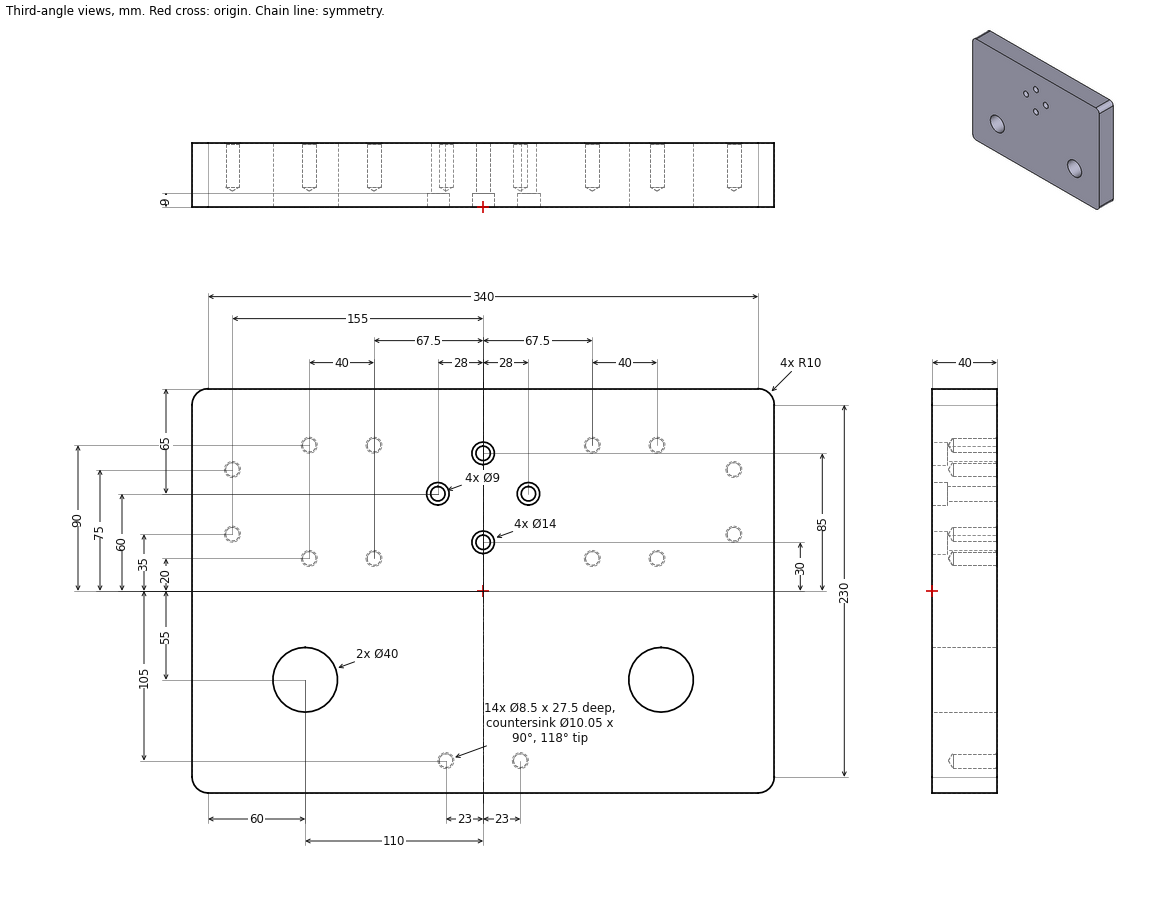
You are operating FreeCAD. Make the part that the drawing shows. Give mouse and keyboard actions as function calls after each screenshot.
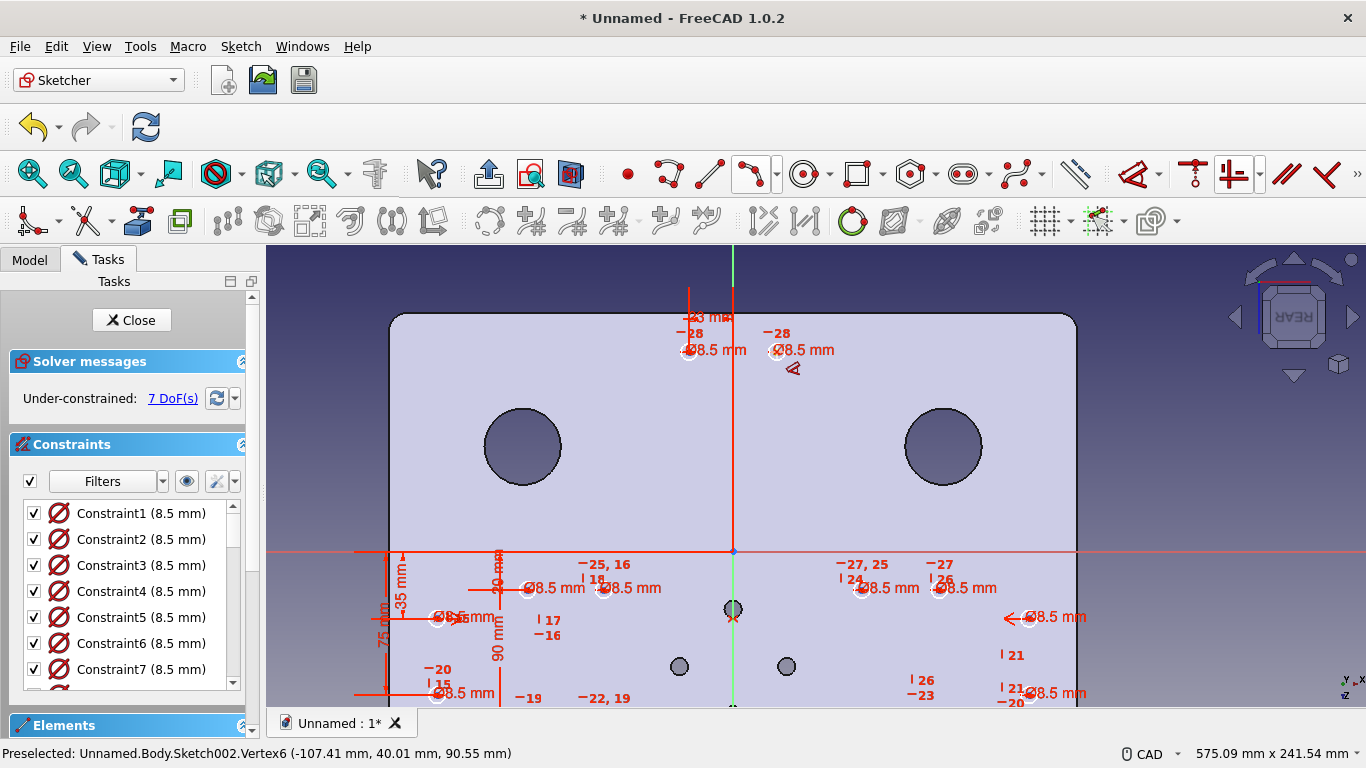
click(777, 352)
click(755, 586)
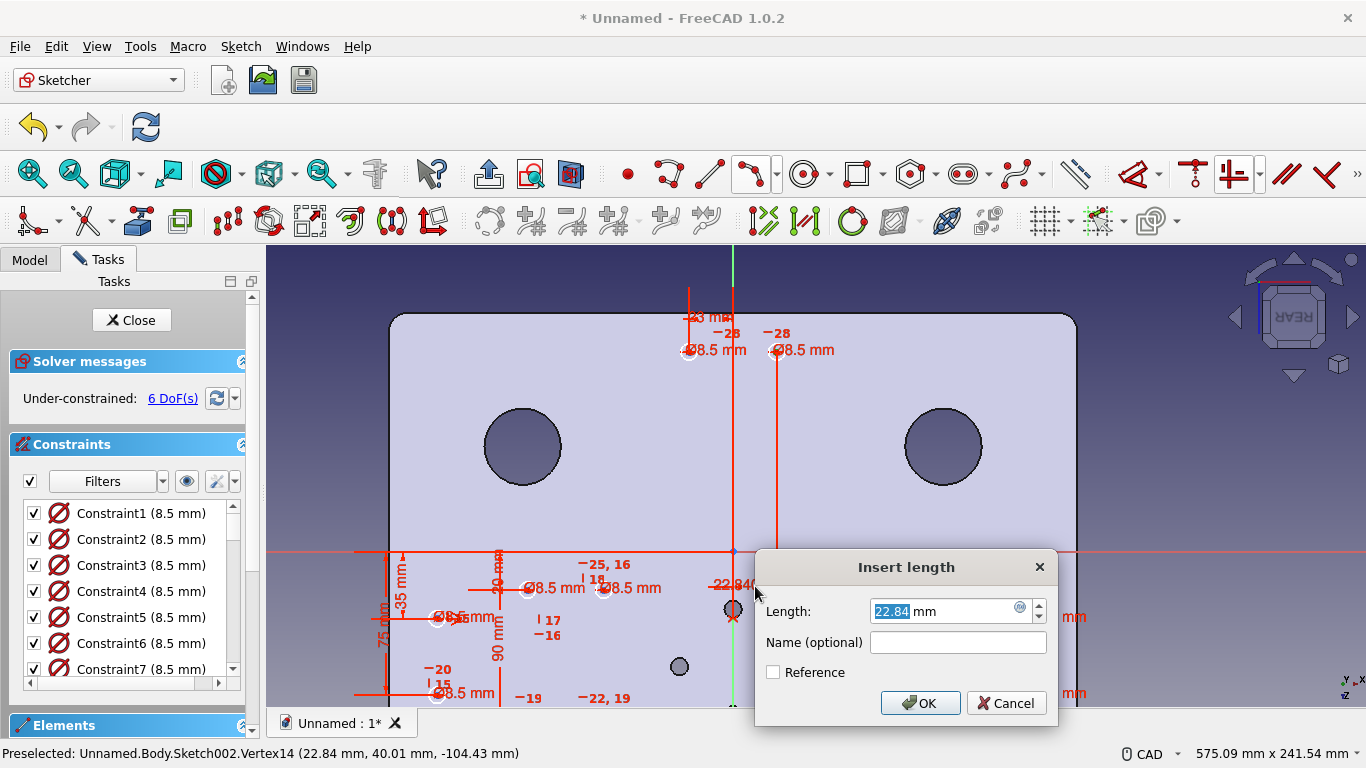
text(23)
key(Return)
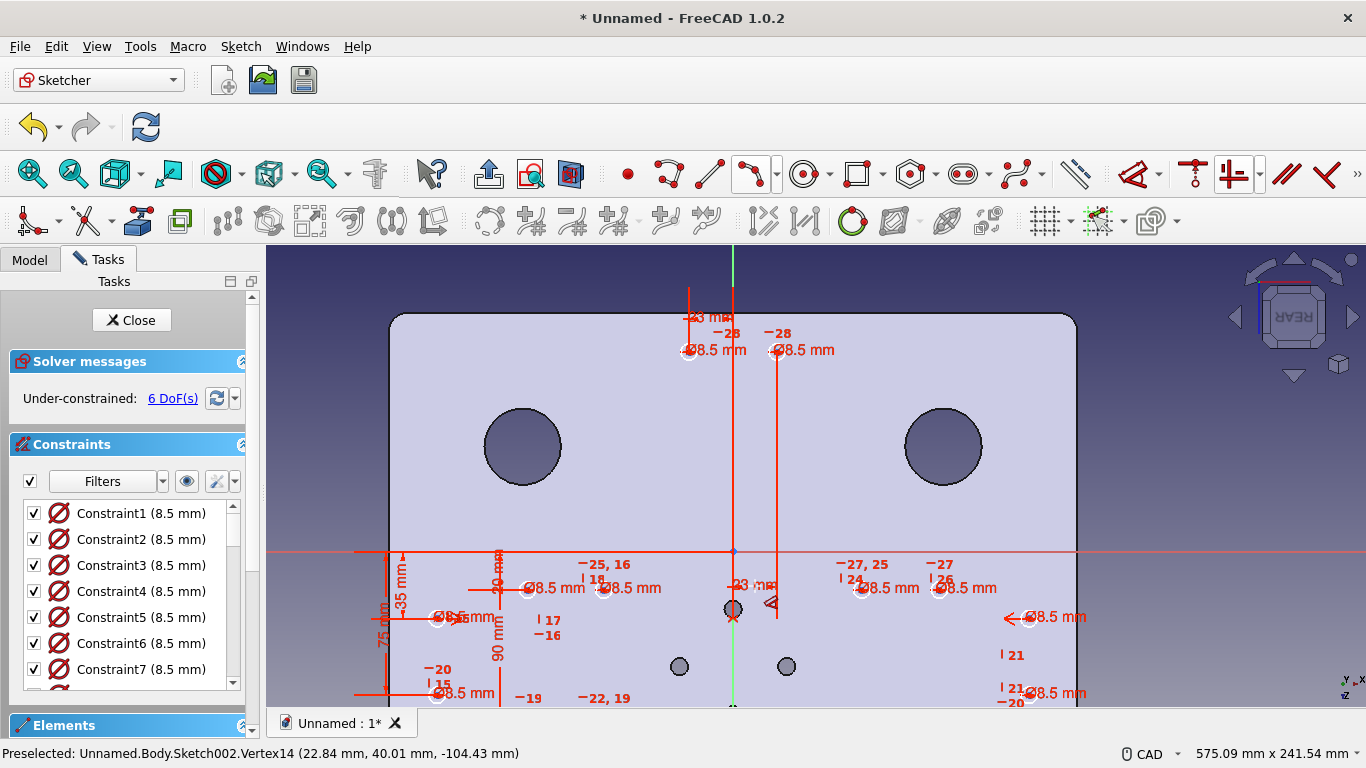
click(689, 352)
click(655, 452)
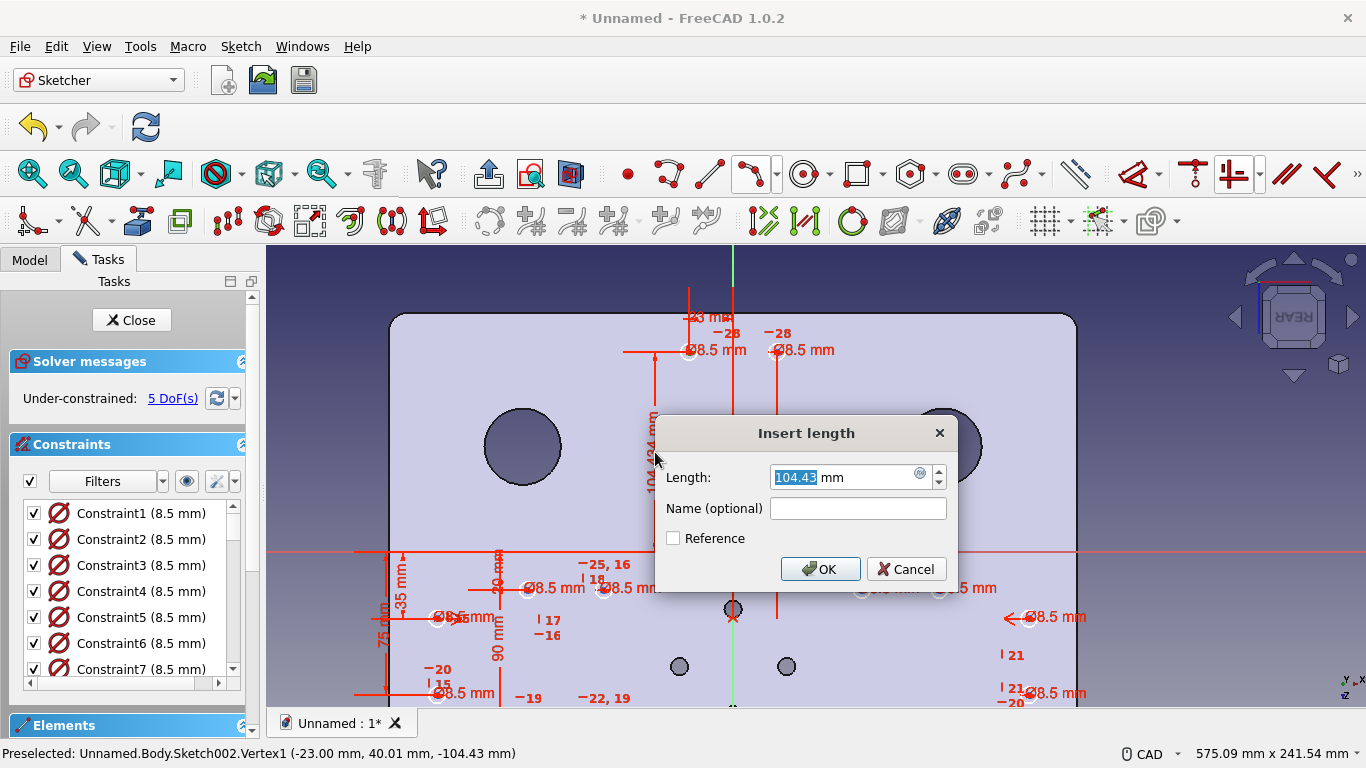
text(105)
key(Return)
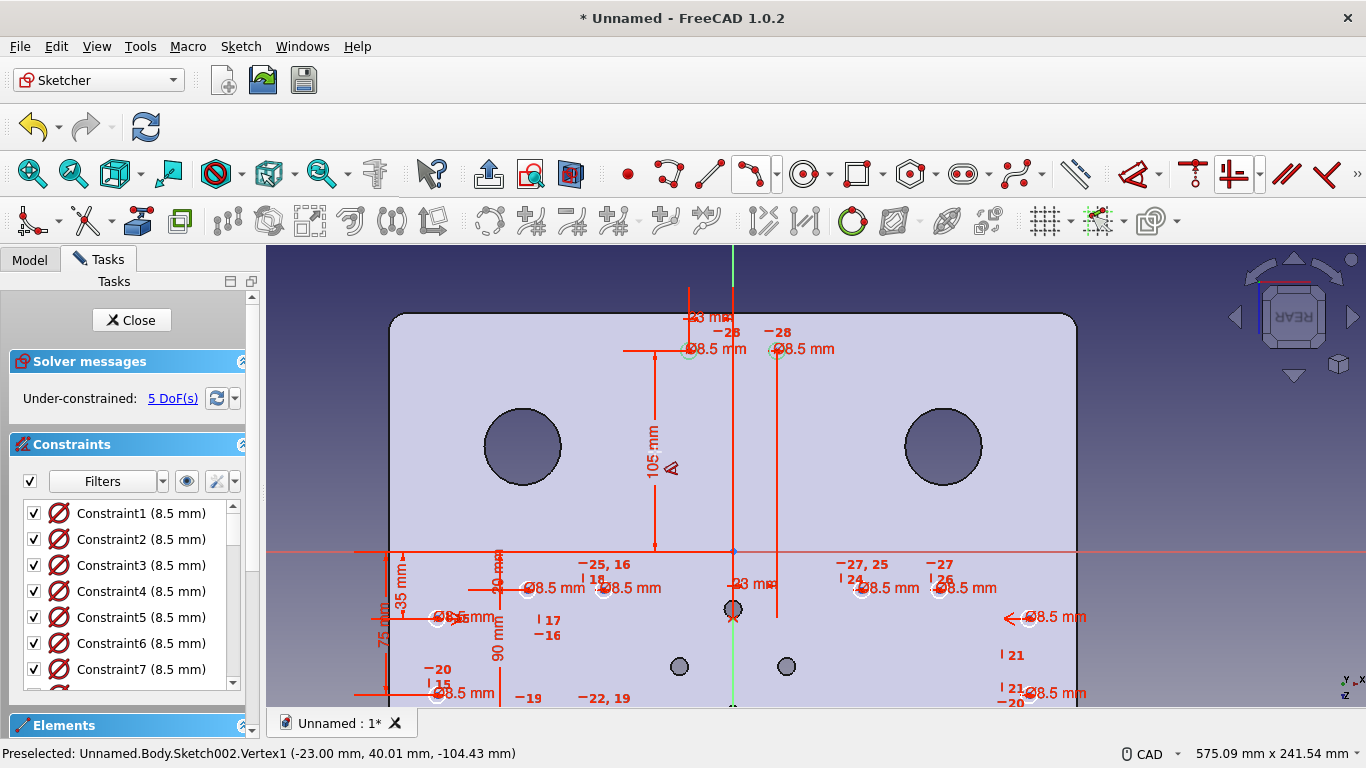
click(437, 619)
click(585, 653)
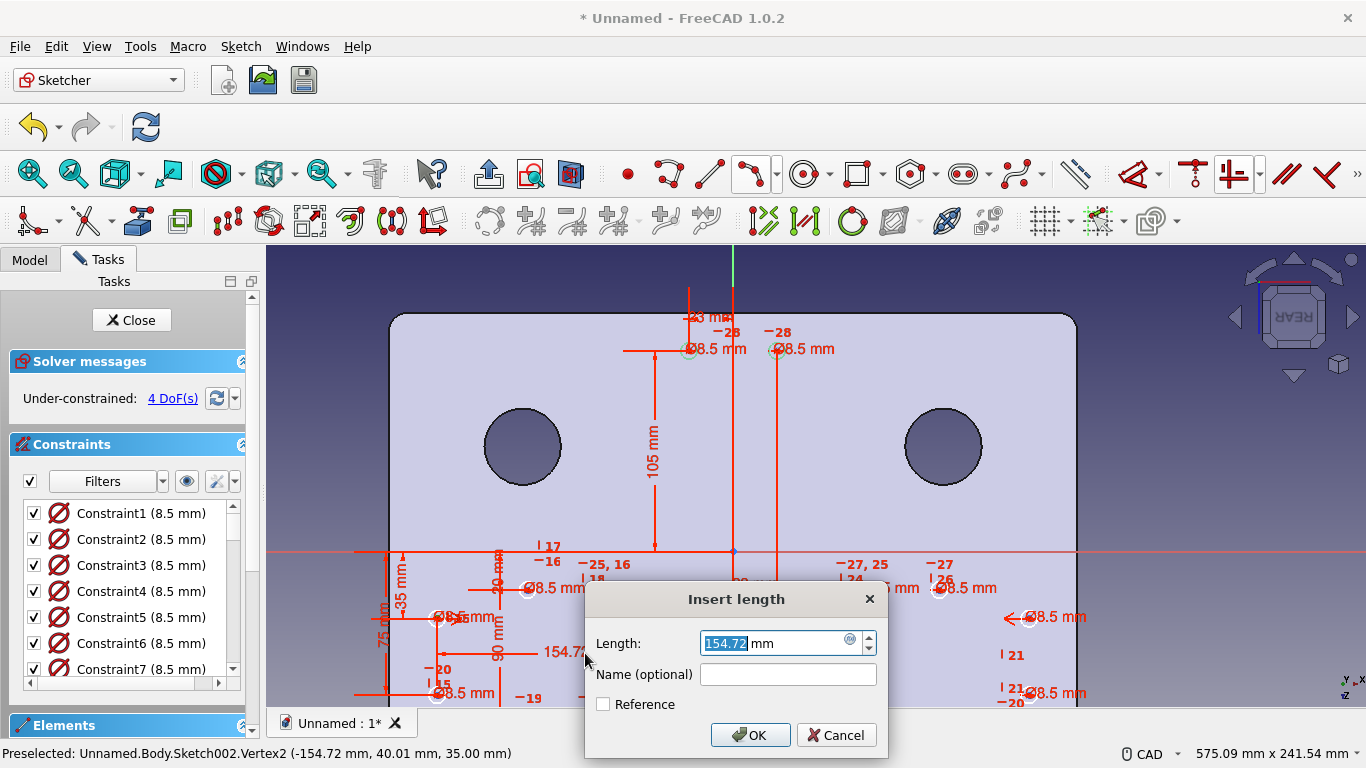
text(155)
key(Return)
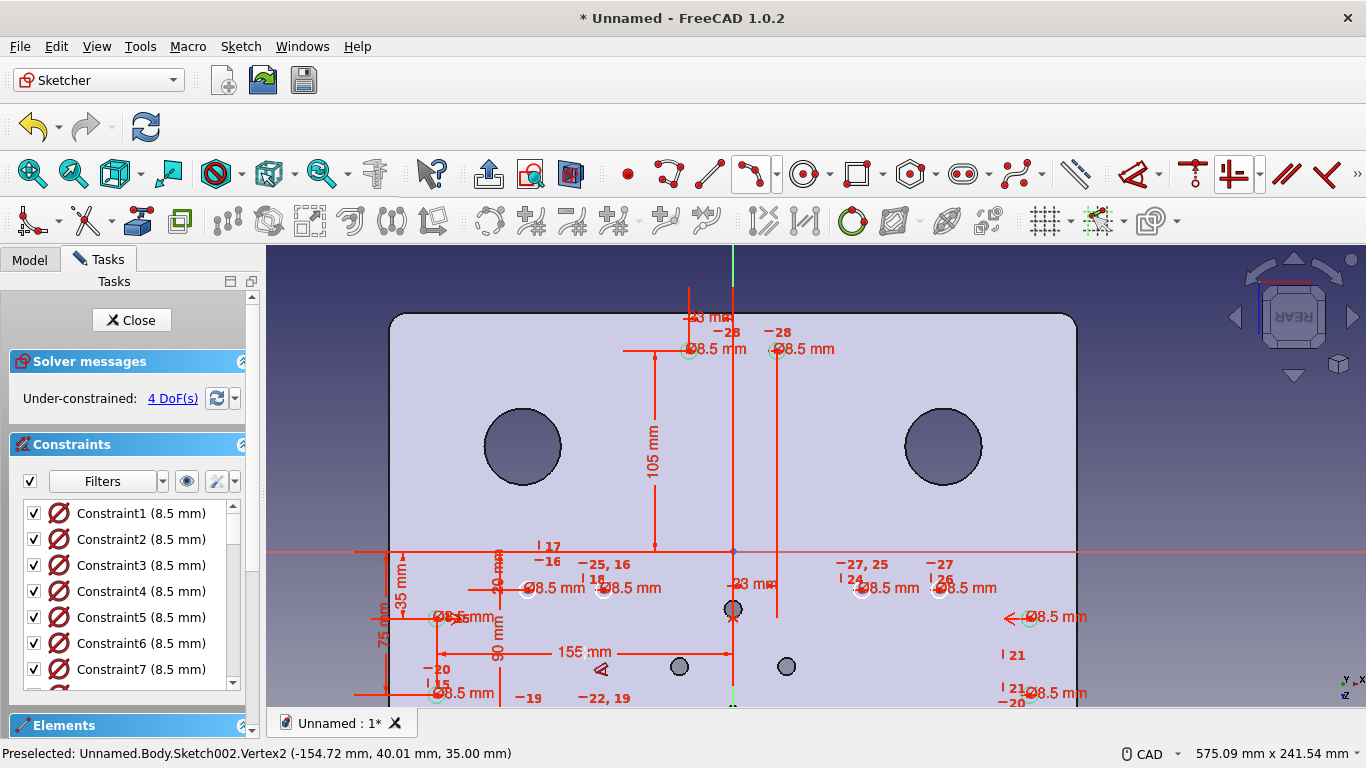
click(528, 590)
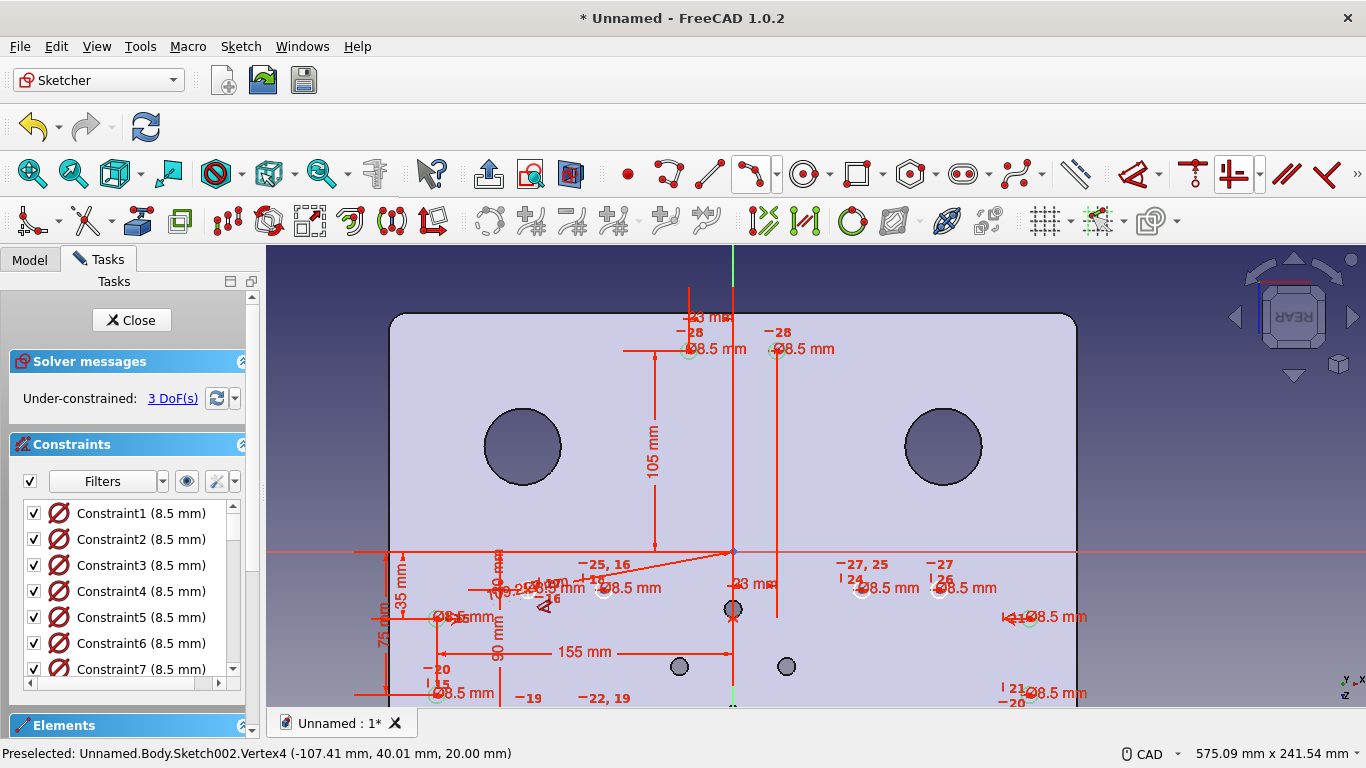
click(604, 590)
click(583, 624)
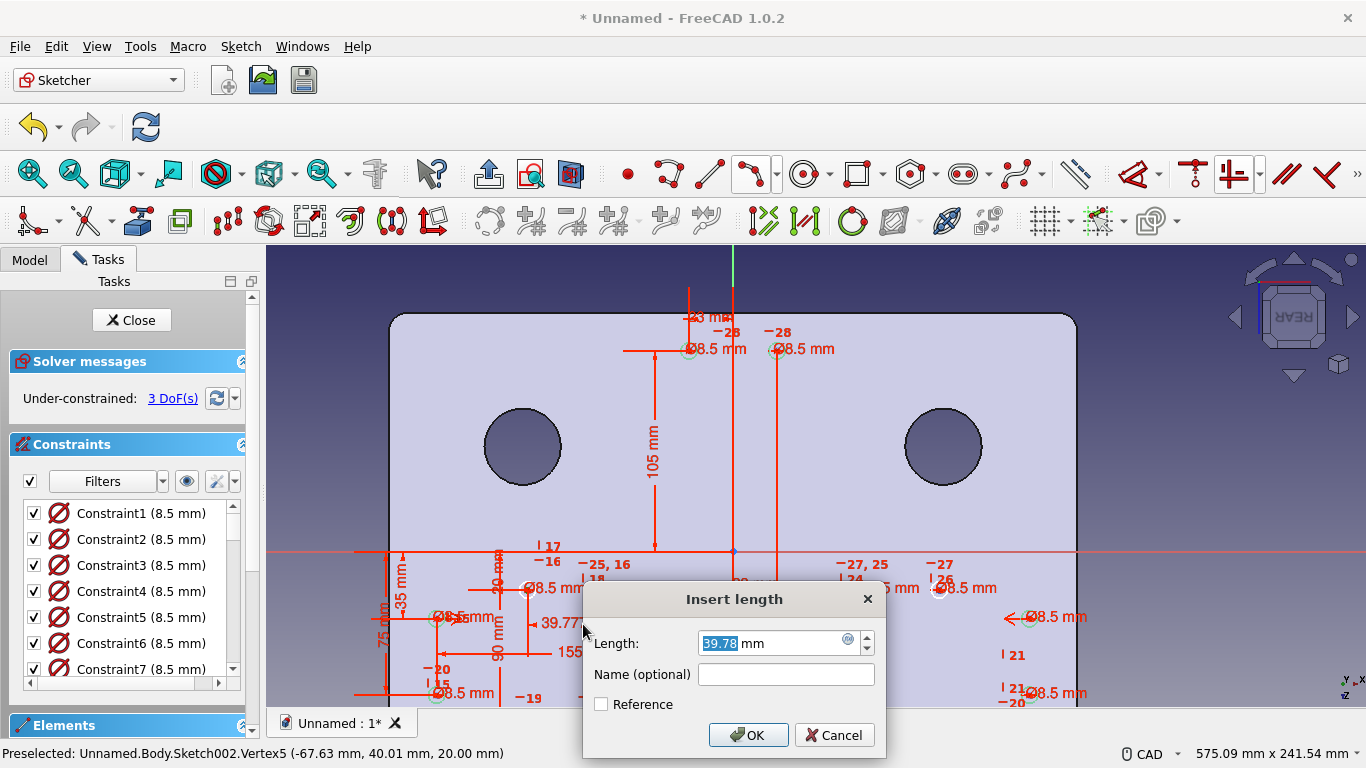
text(40)
key(Return)